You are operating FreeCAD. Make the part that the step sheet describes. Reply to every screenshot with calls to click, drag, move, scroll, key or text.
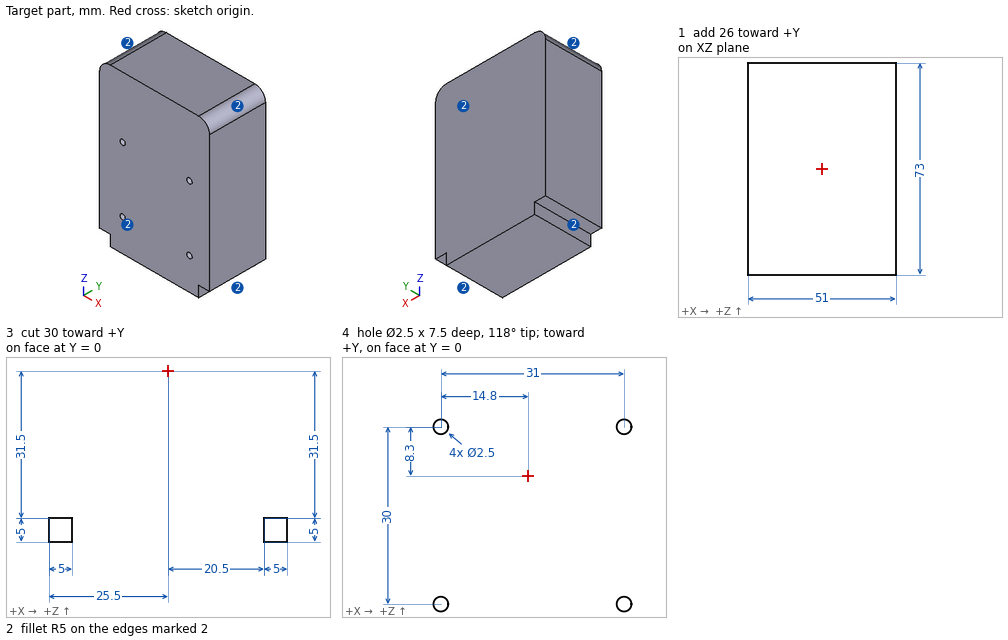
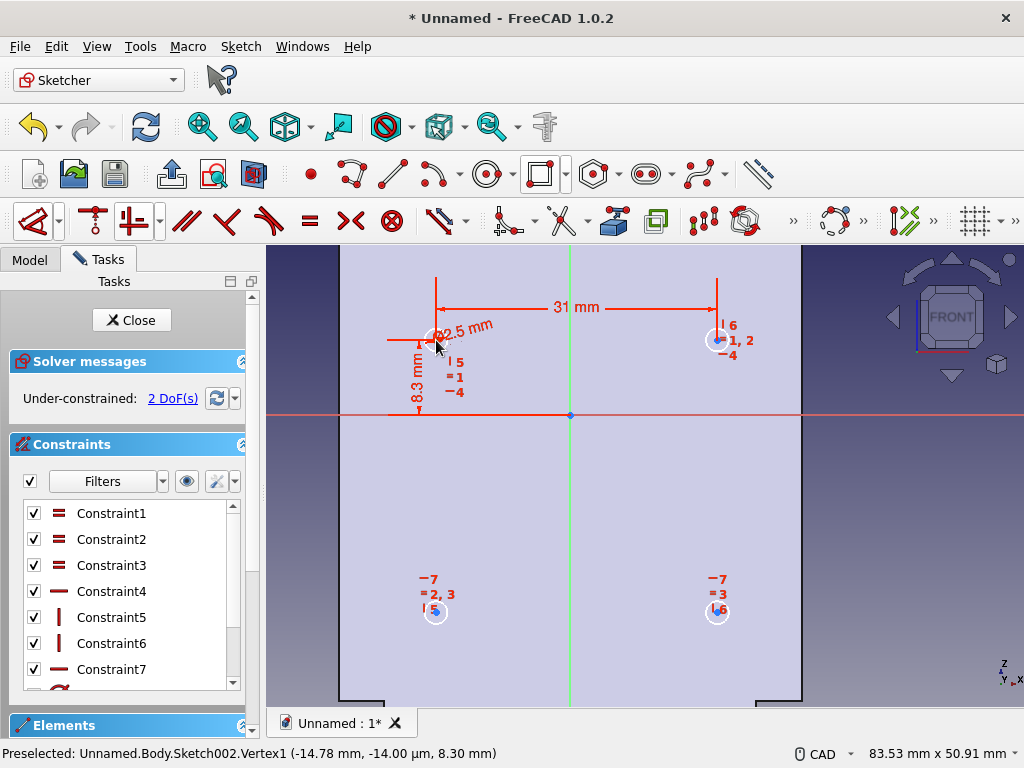
click(436, 613)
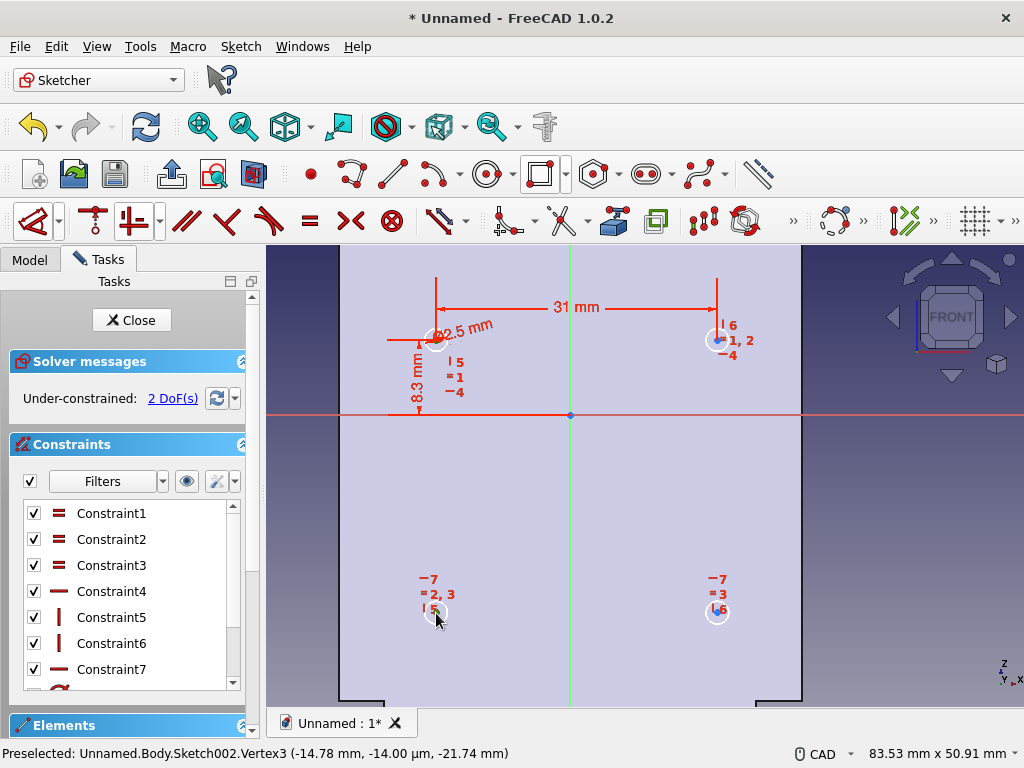
click(58, 222)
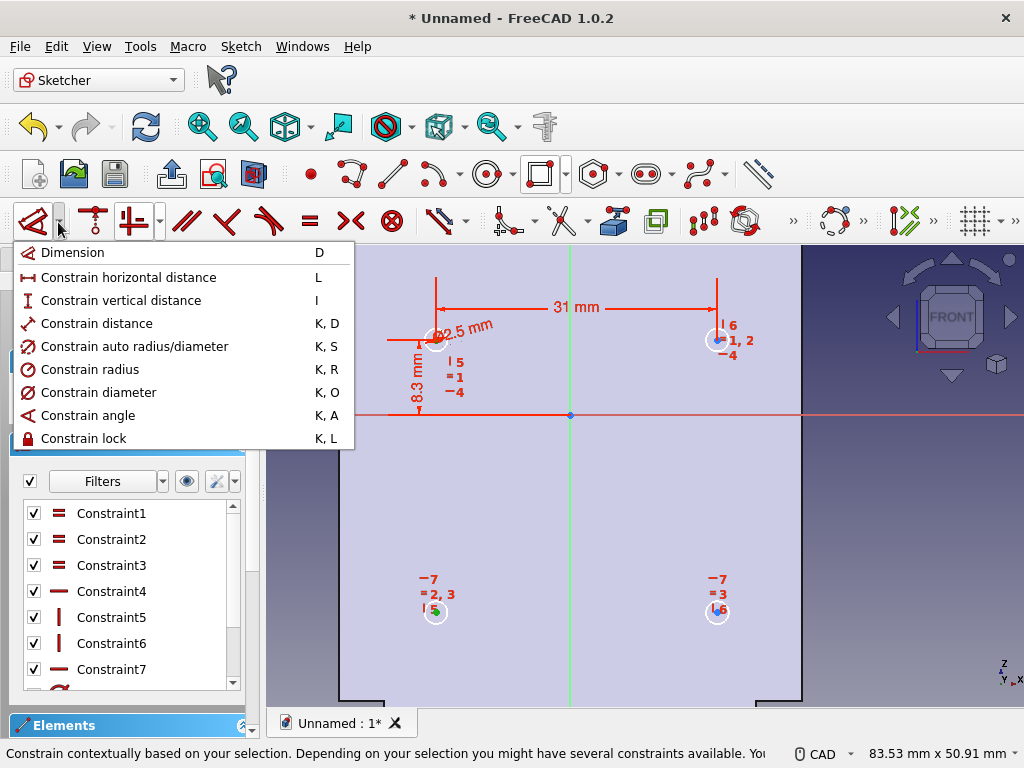
click(184, 300)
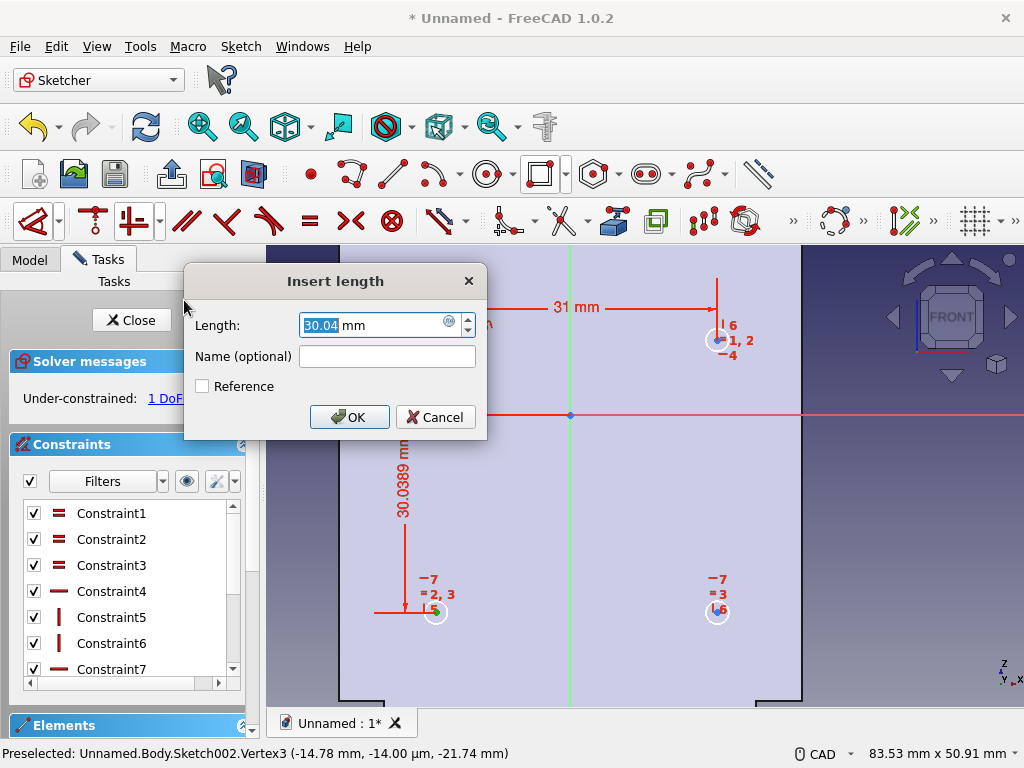
text(30)
key(Return)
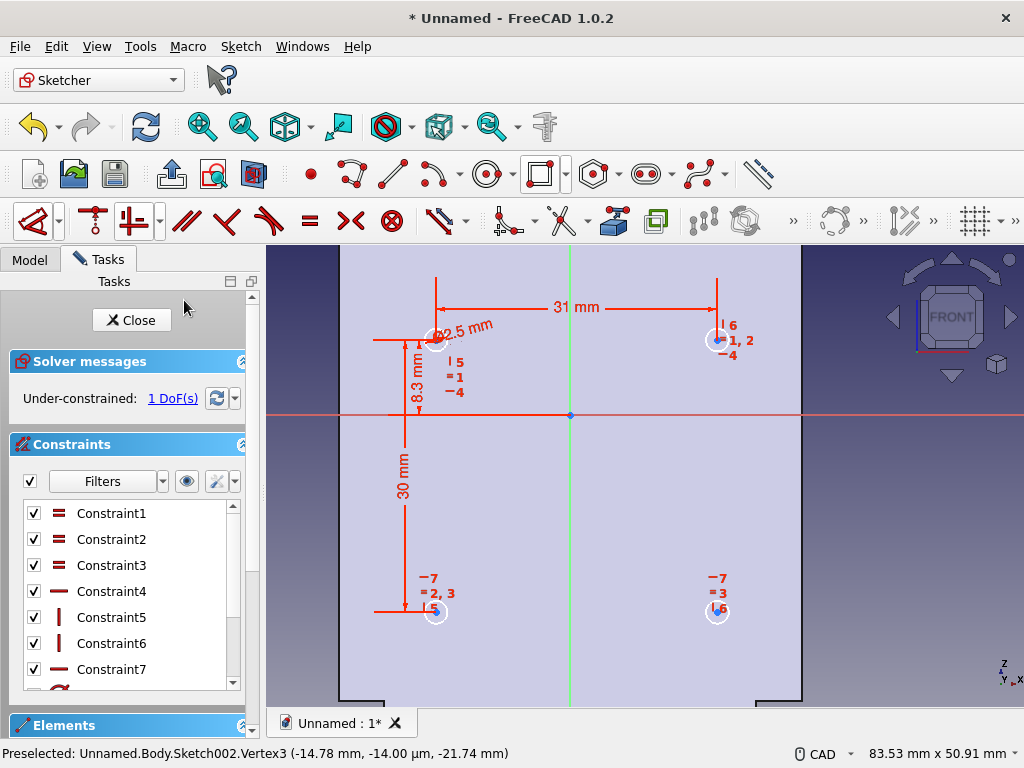
click(436, 340)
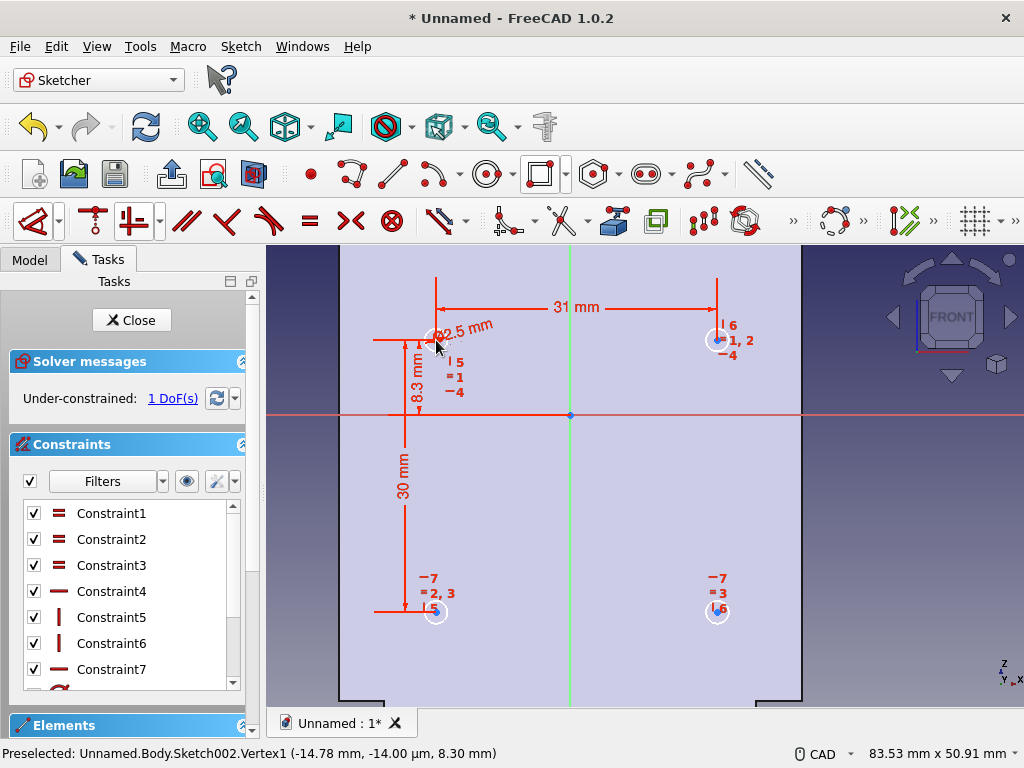
click(58, 222)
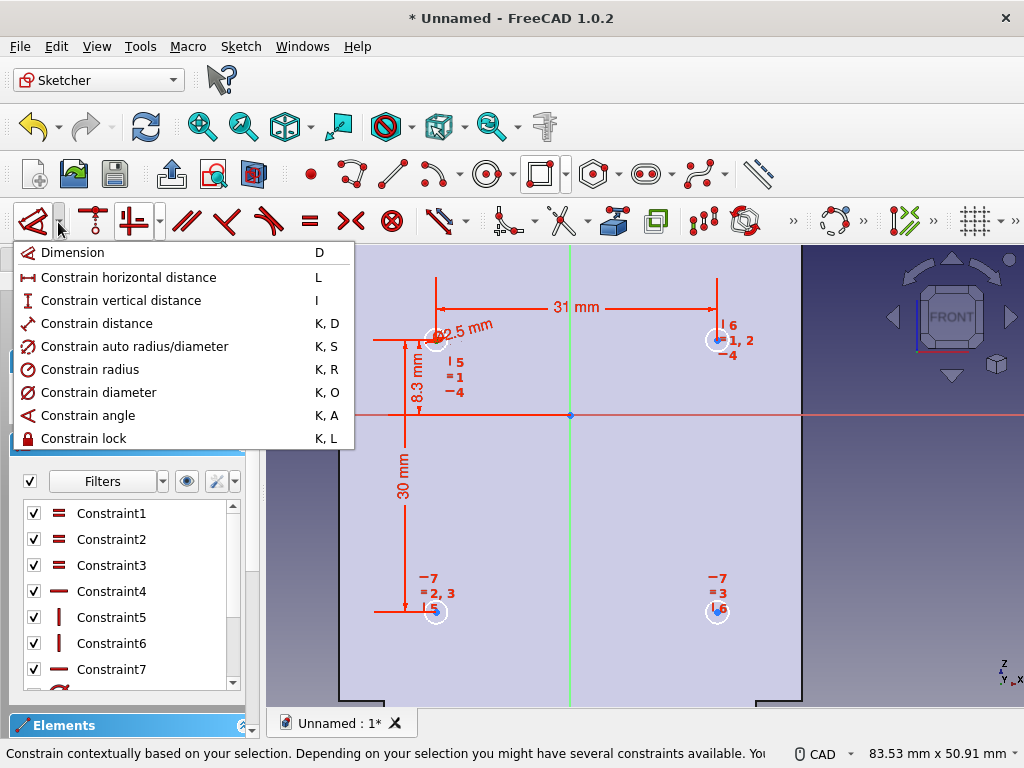
click(184, 278)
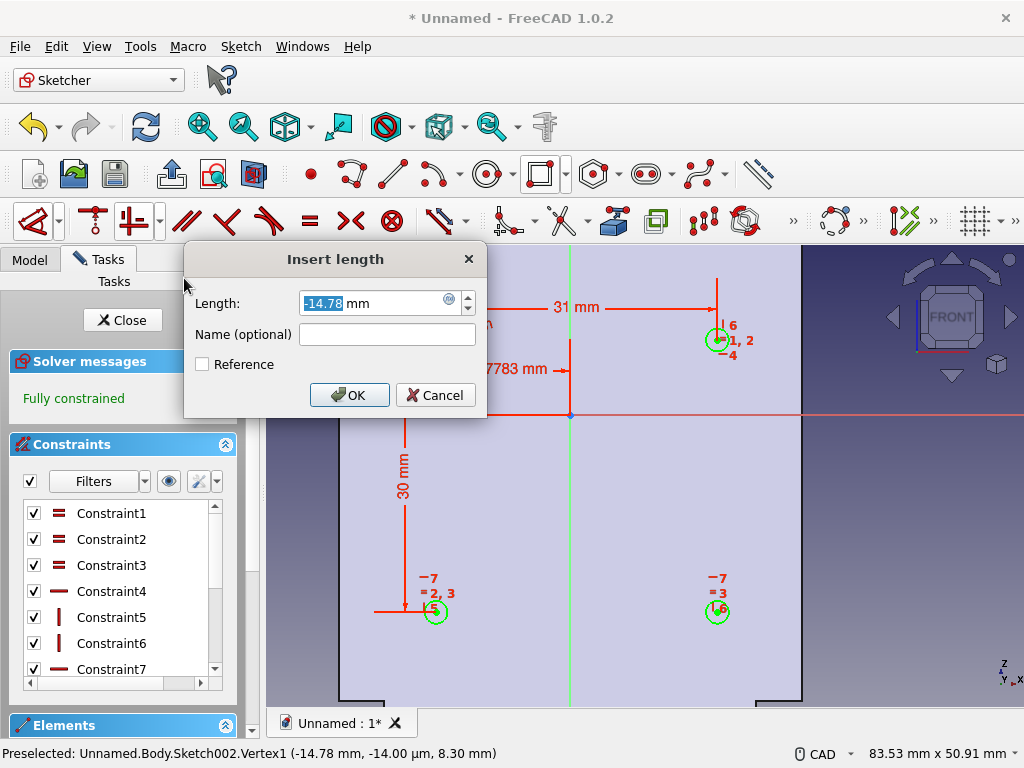
text(-14.8)
key(Return)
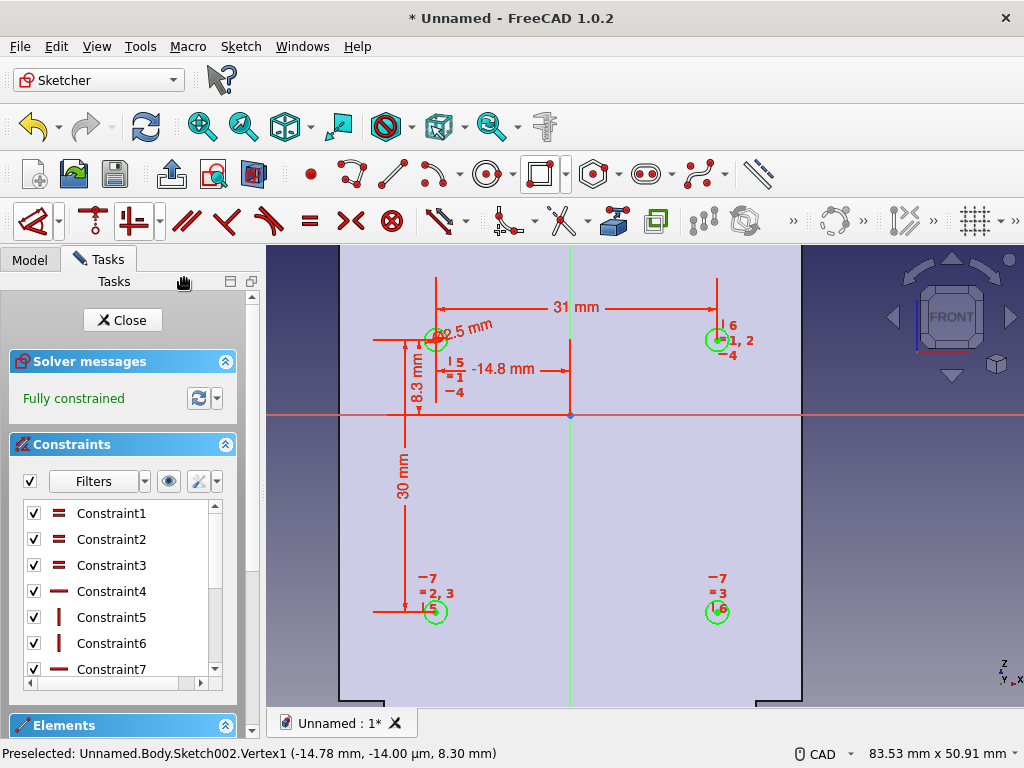
click(123, 320)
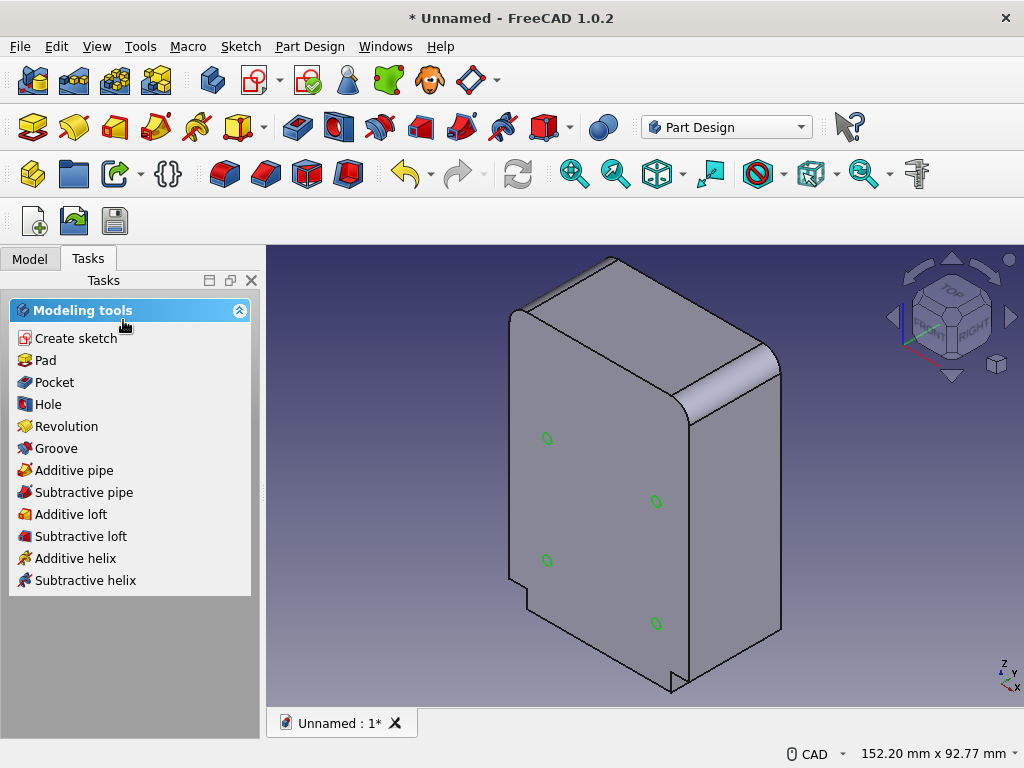
click(339, 128)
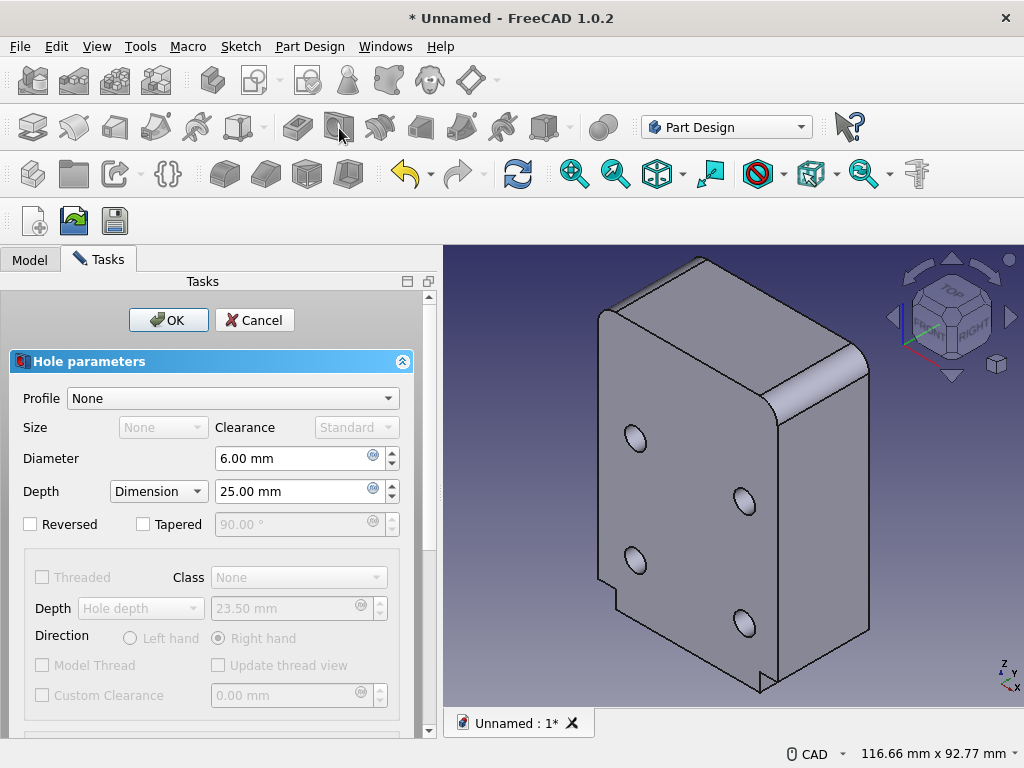
triple_click(300, 458)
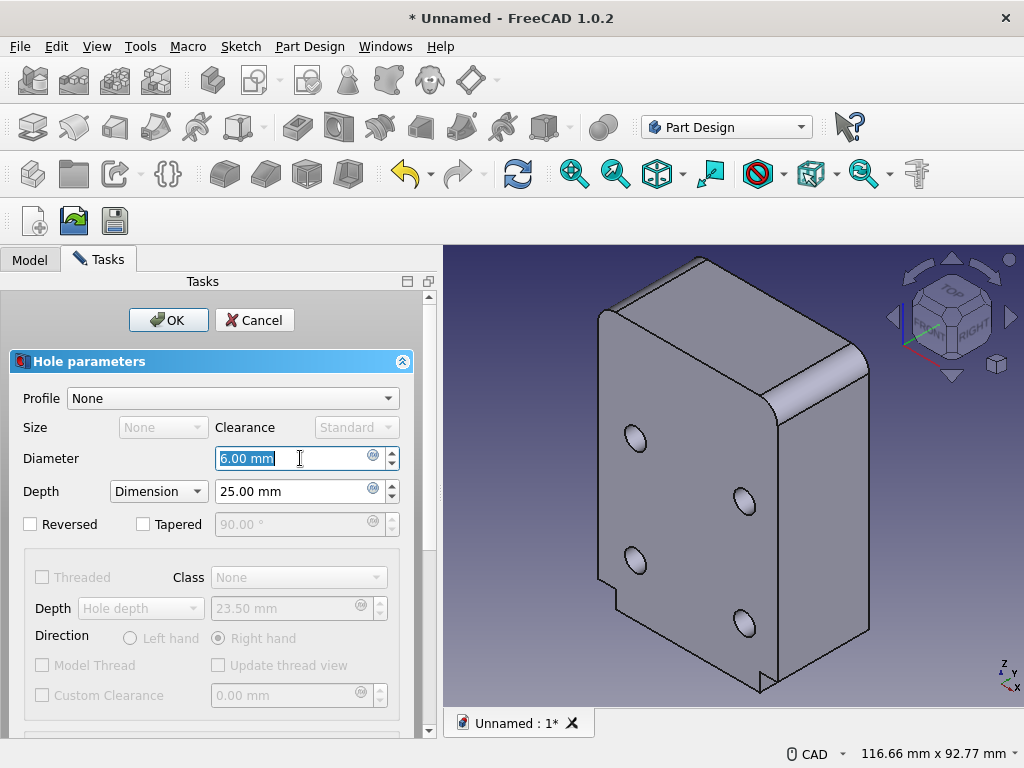
text(2.5)
key(Tab)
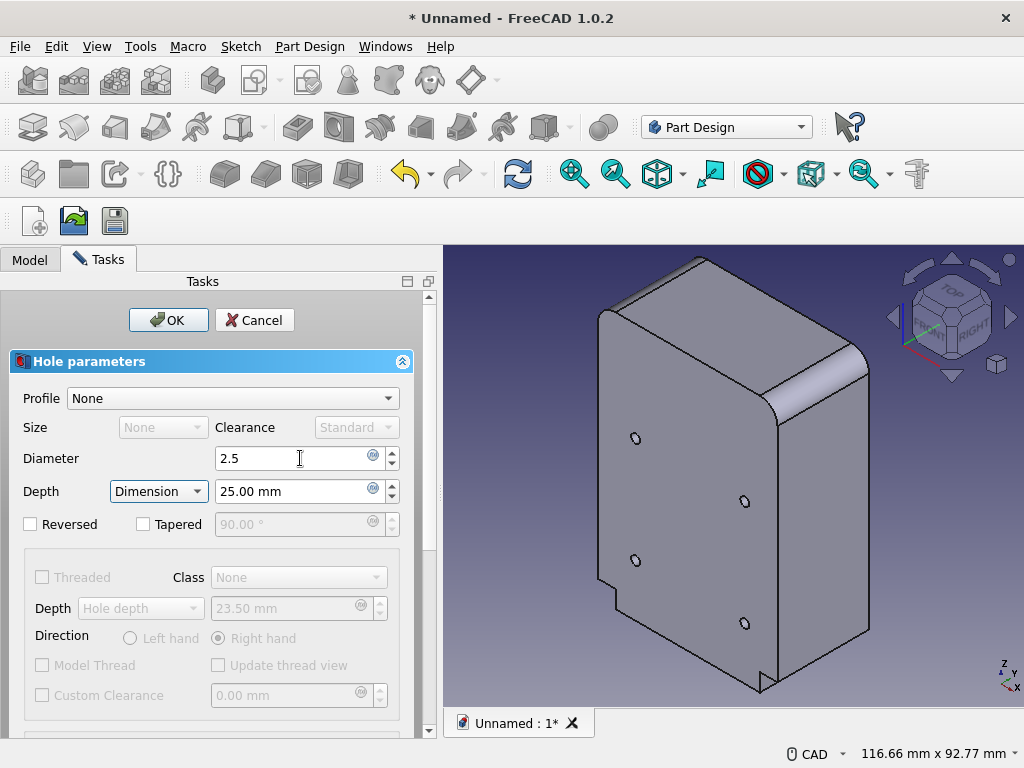
triple_click(300, 492)